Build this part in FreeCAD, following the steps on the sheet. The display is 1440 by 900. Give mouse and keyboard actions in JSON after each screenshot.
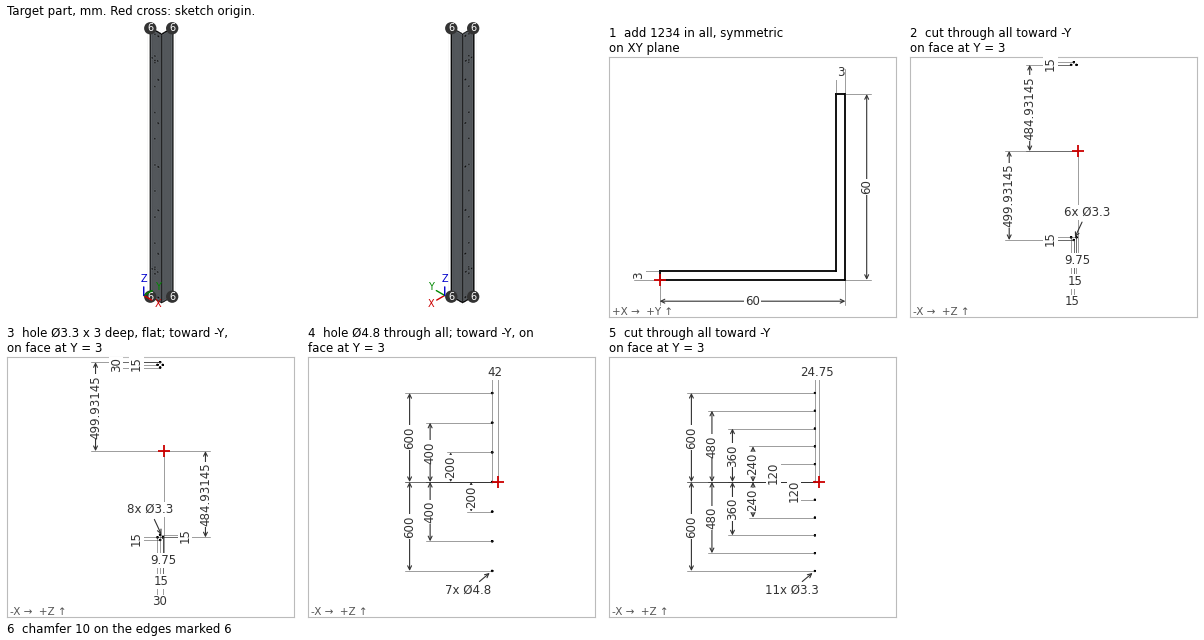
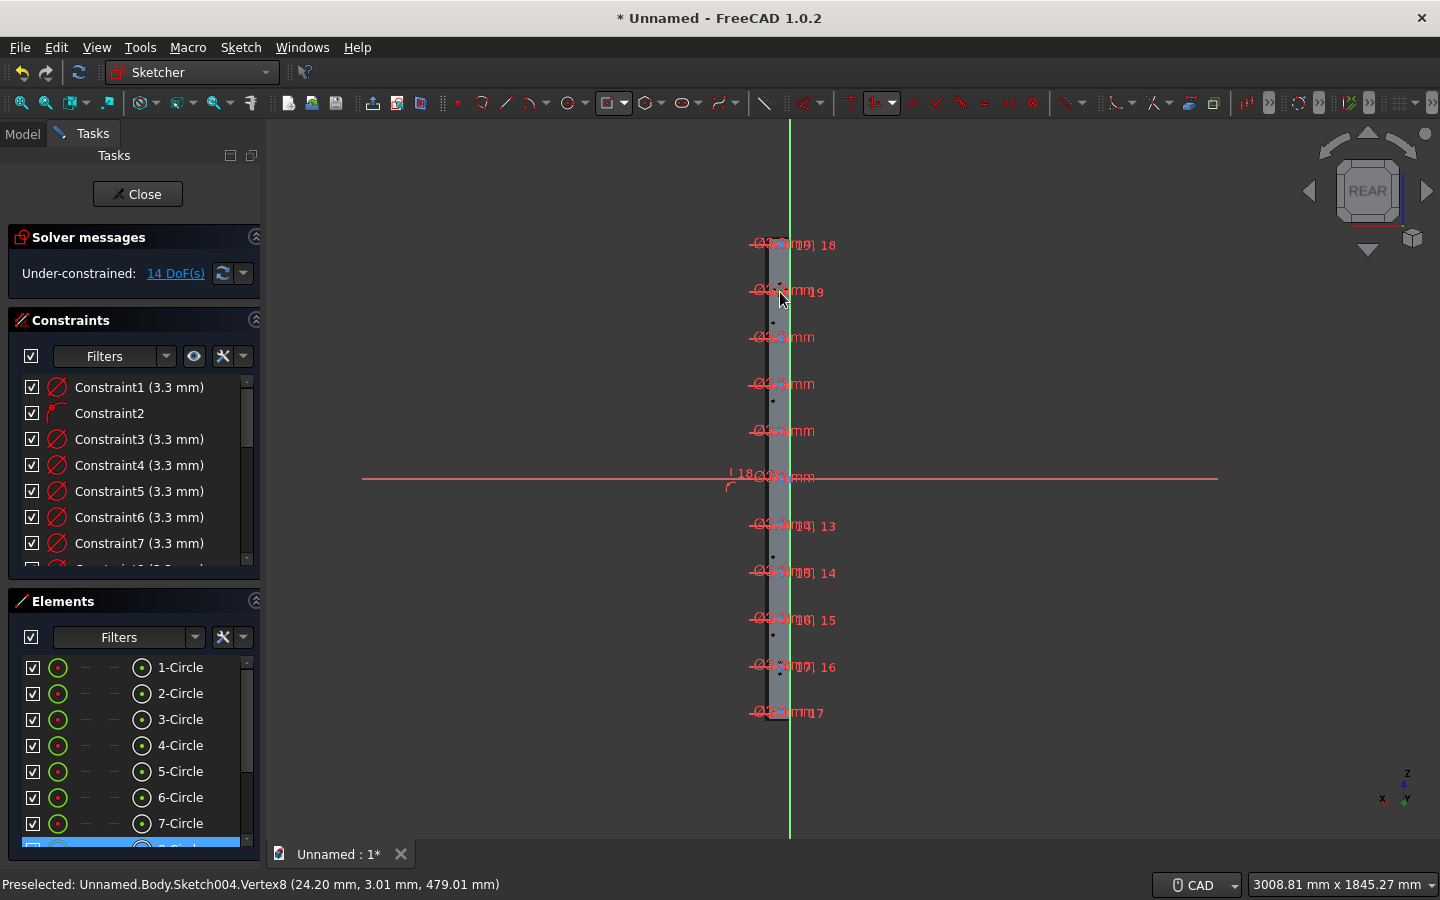
{"action": "left_click", "coordinate": [780, 339]}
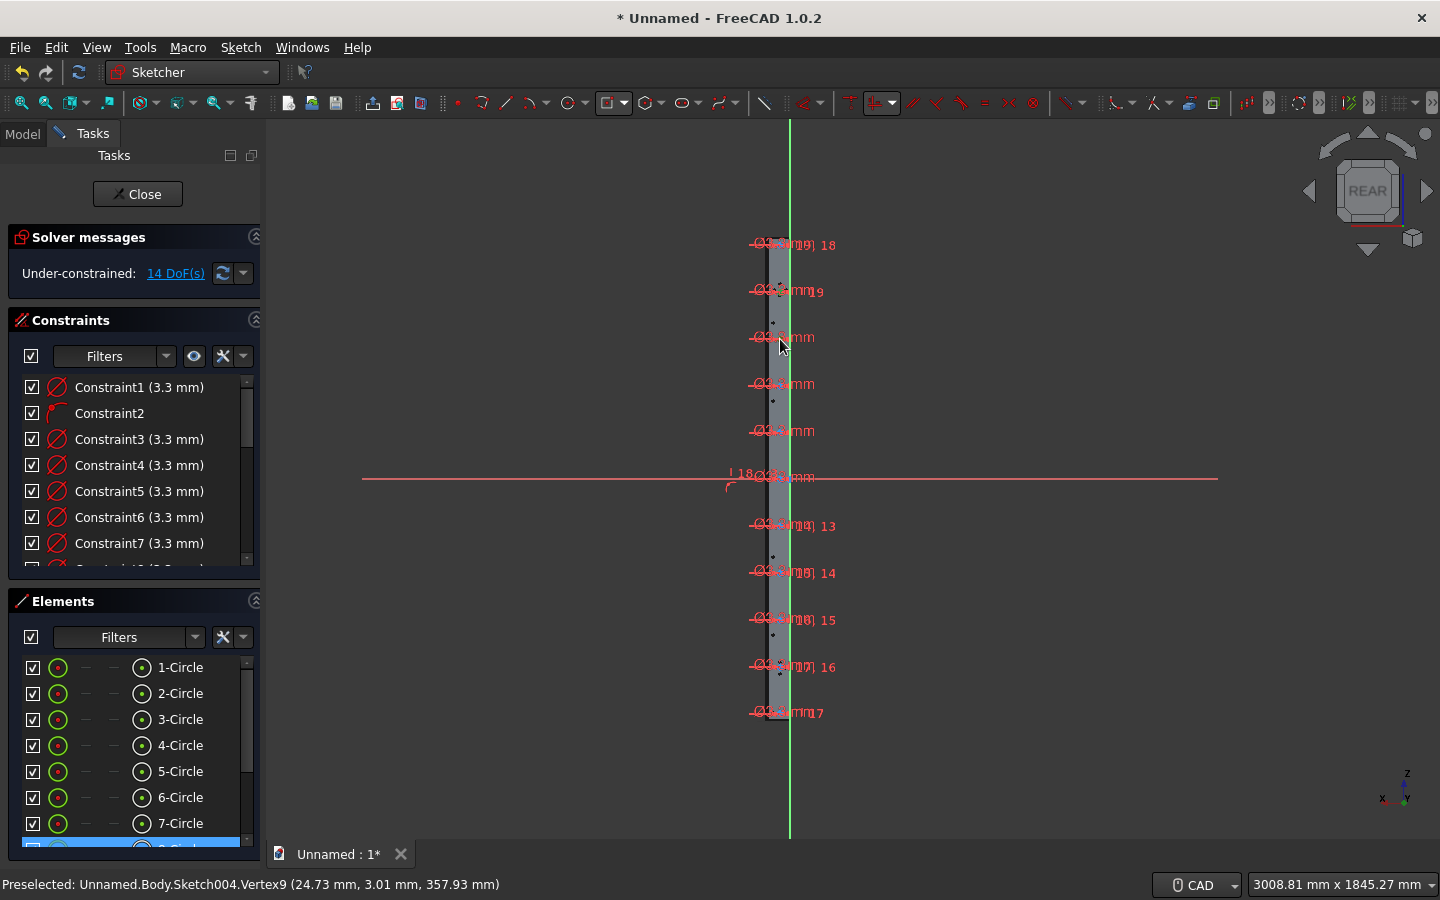
{"action": "left_click", "coordinate": [894, 104]}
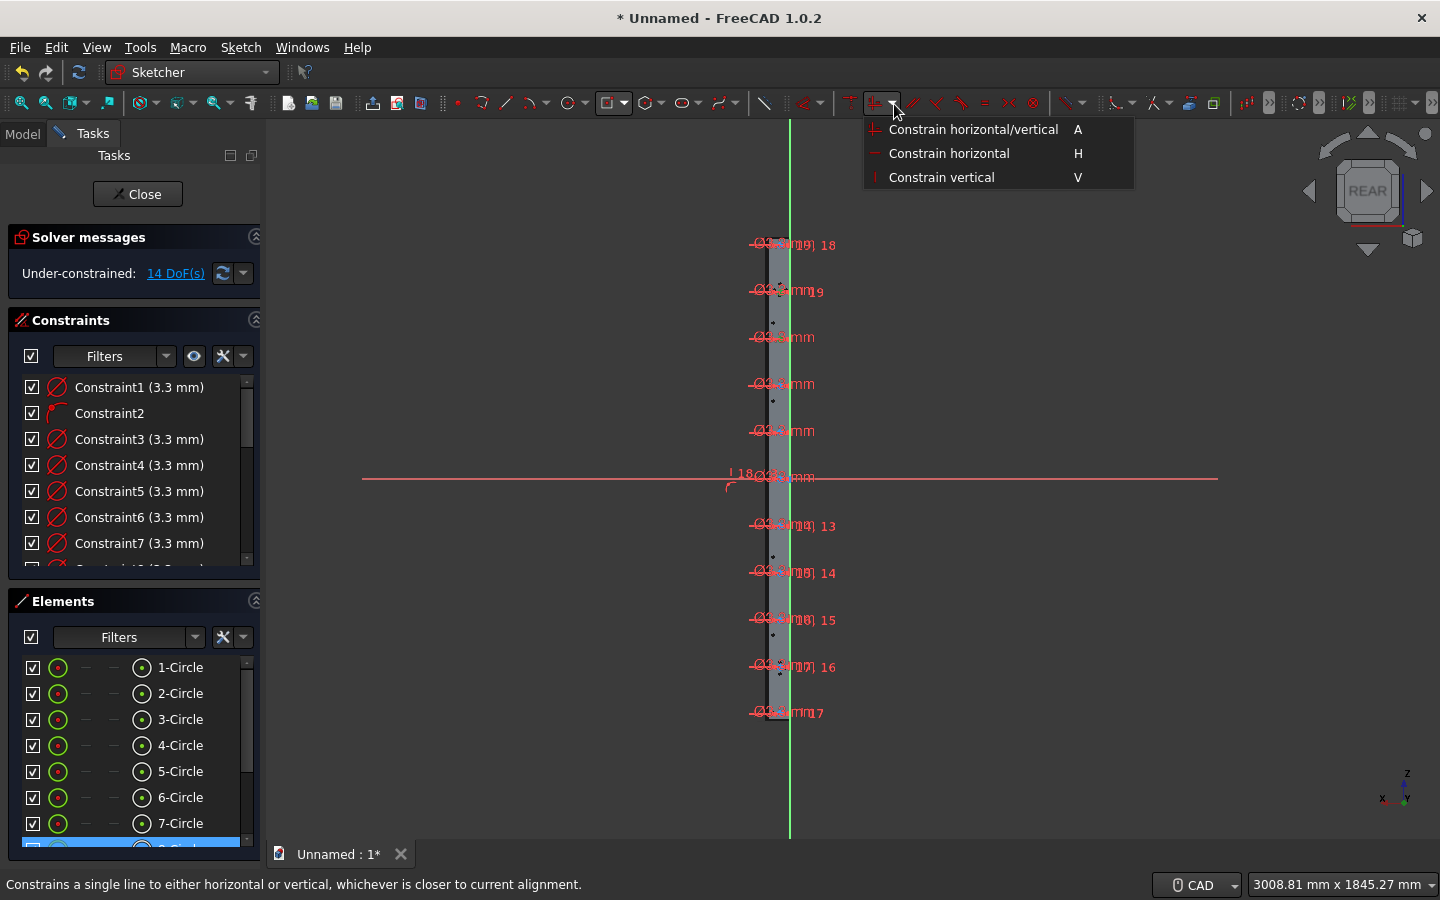
{"action": "left_click", "coordinate": [999, 177]}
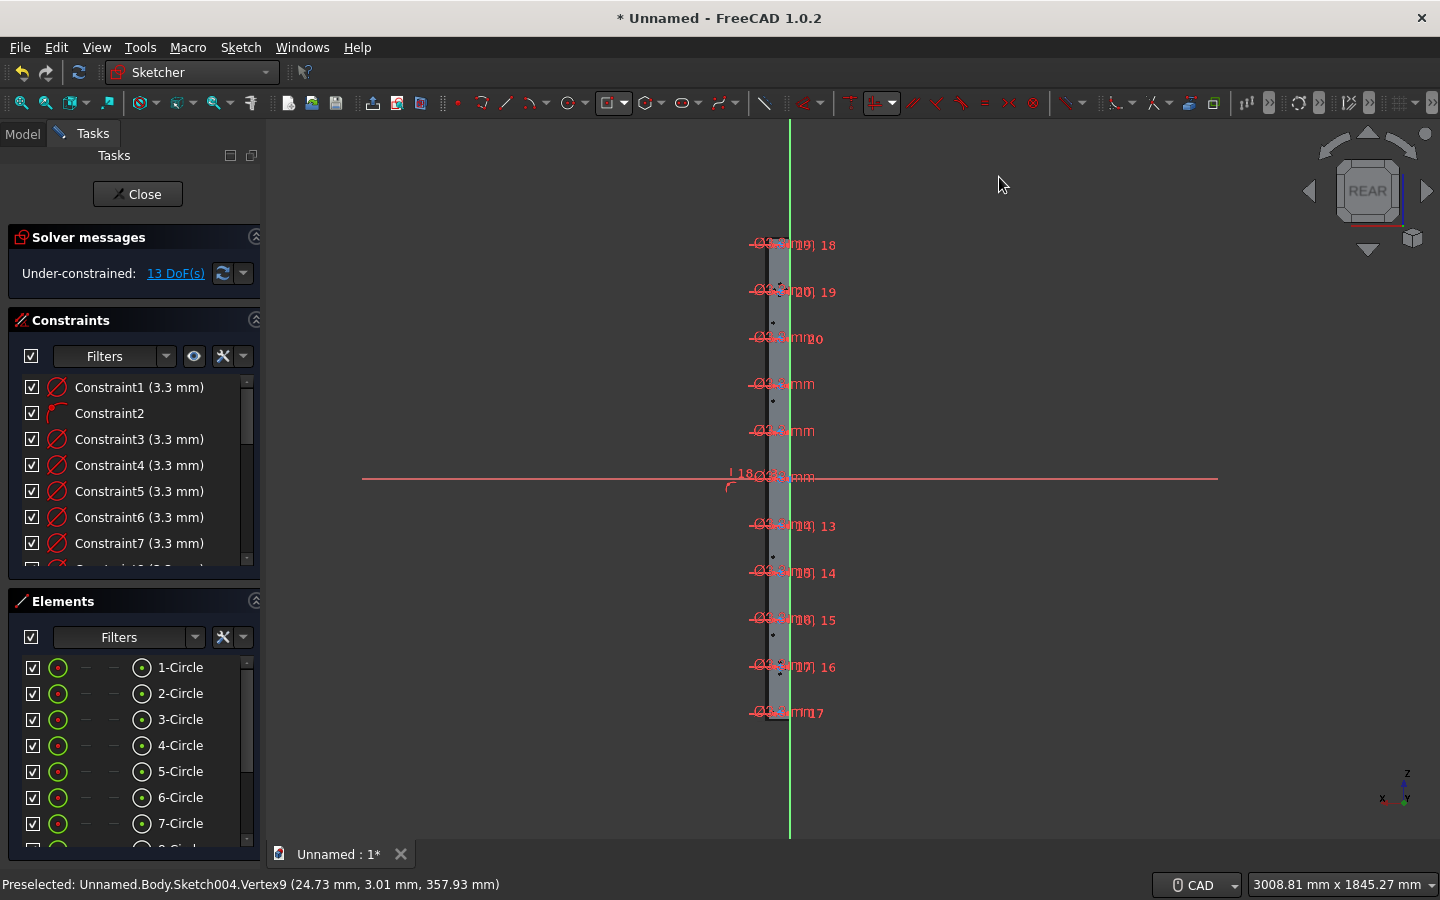
{"action": "left_click", "coordinate": [780, 339]}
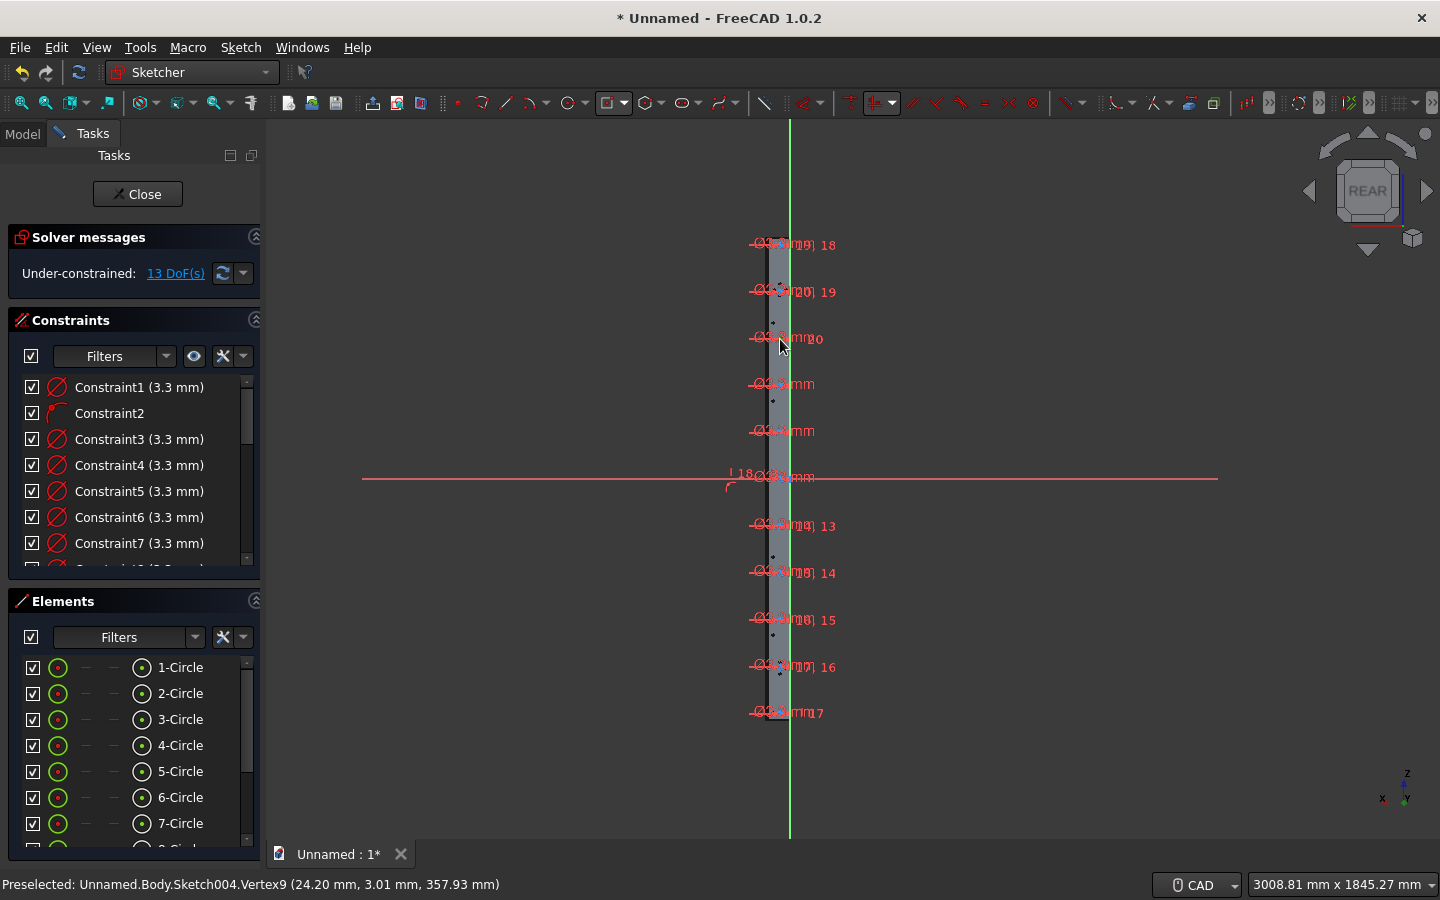
{"action": "left_click", "coordinate": [780, 386]}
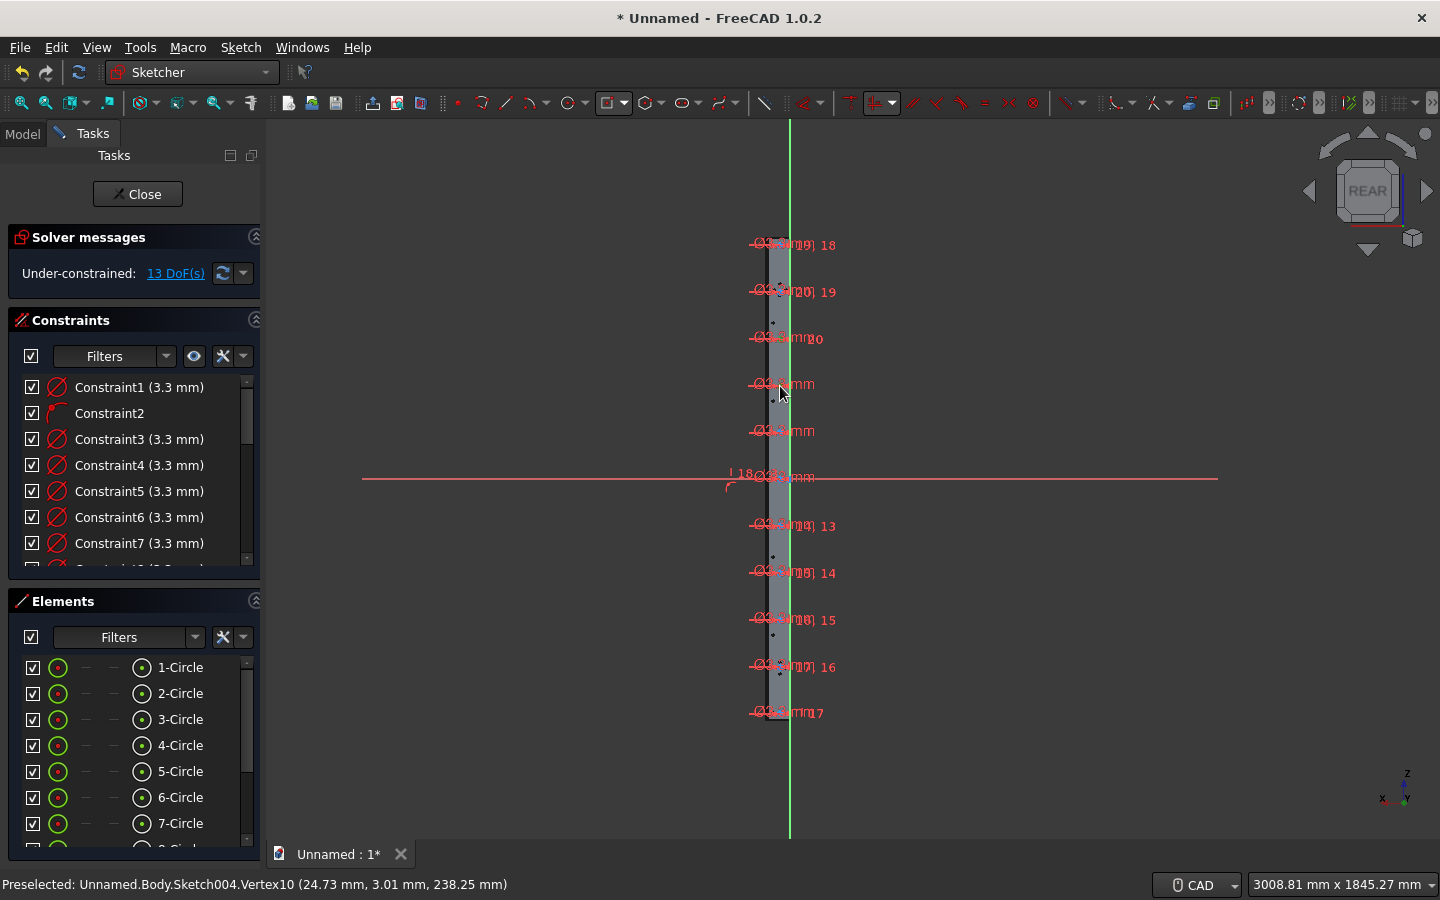
{"action": "left_click", "coordinate": [894, 104]}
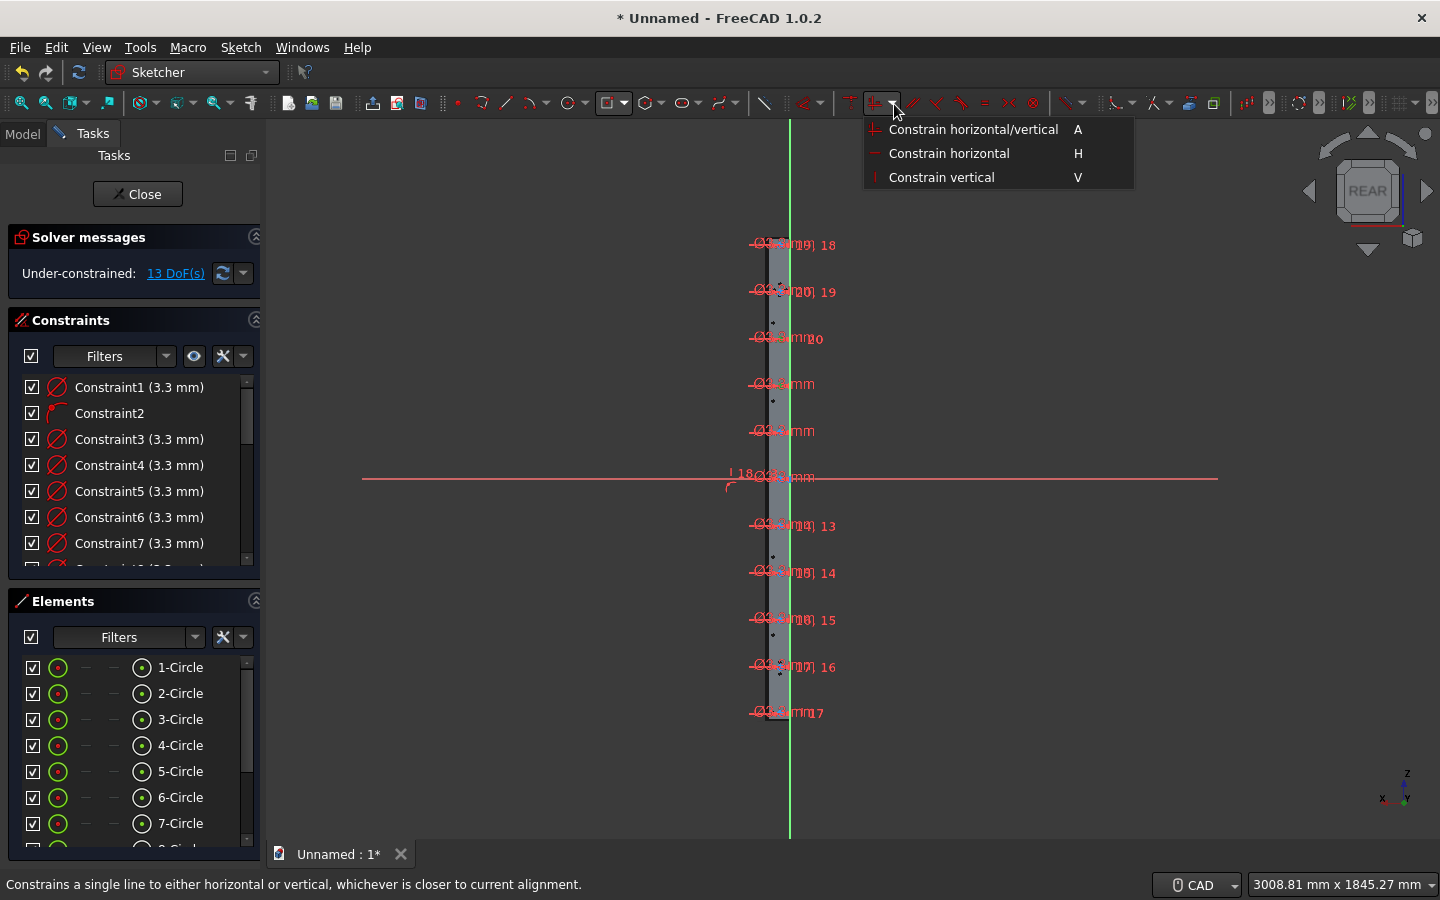
{"action": "left_click", "coordinate": [999, 177]}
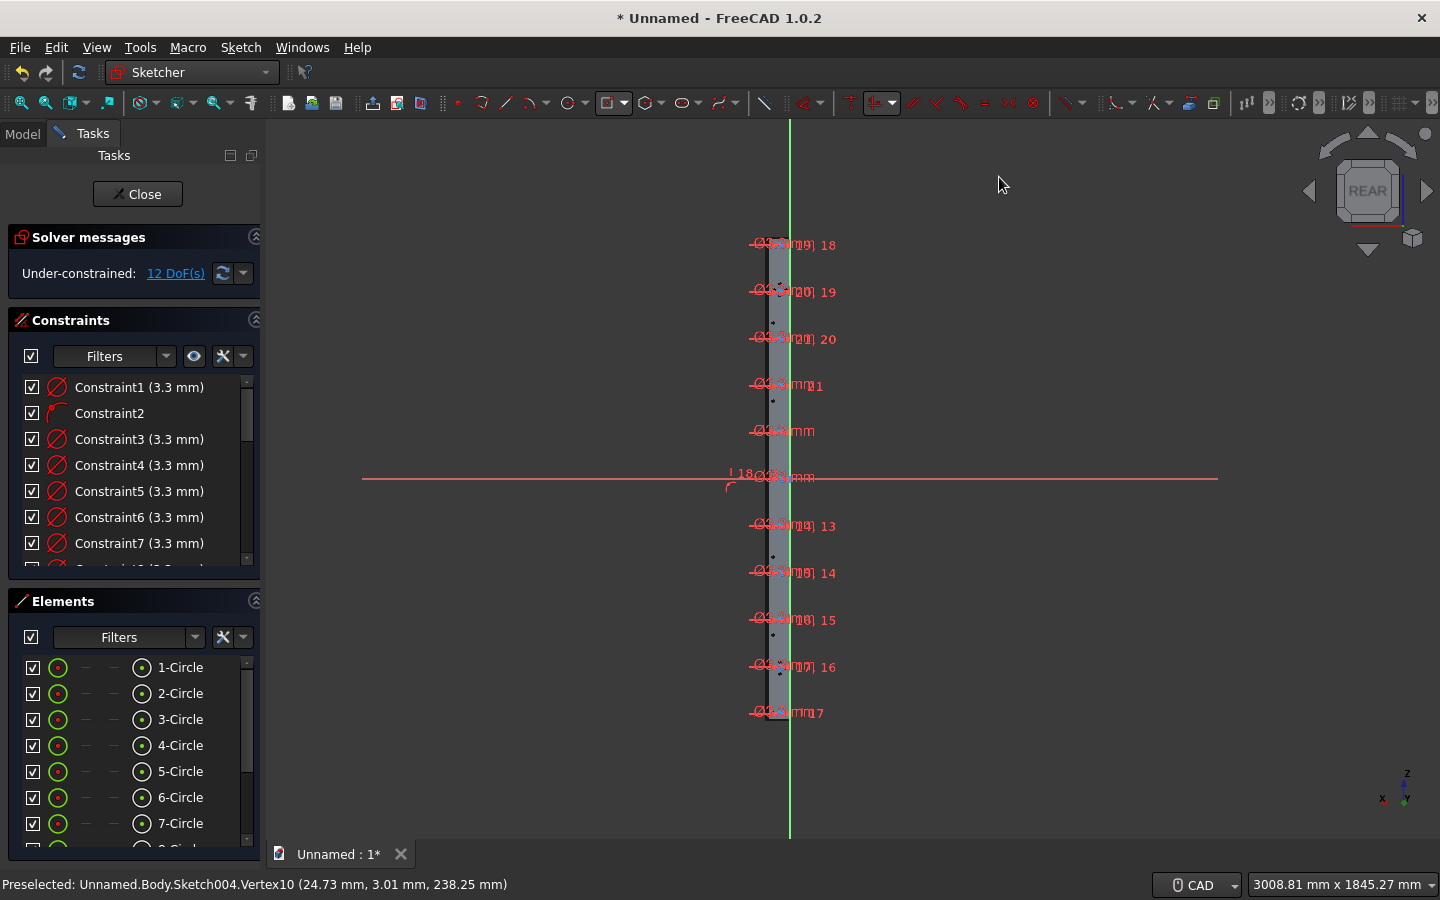
{"action": "scroll", "coordinate": [780, 479], "scroll_direction": "up", "scroll_amount": 2}